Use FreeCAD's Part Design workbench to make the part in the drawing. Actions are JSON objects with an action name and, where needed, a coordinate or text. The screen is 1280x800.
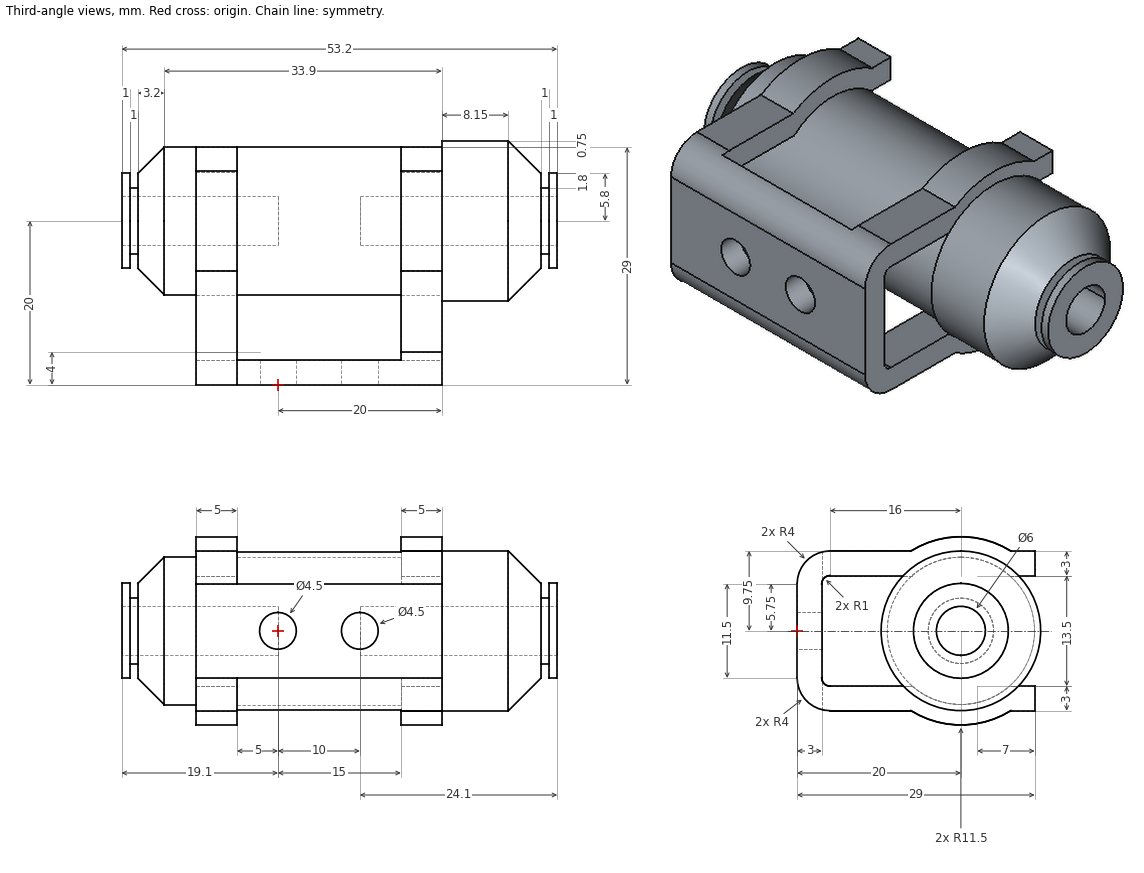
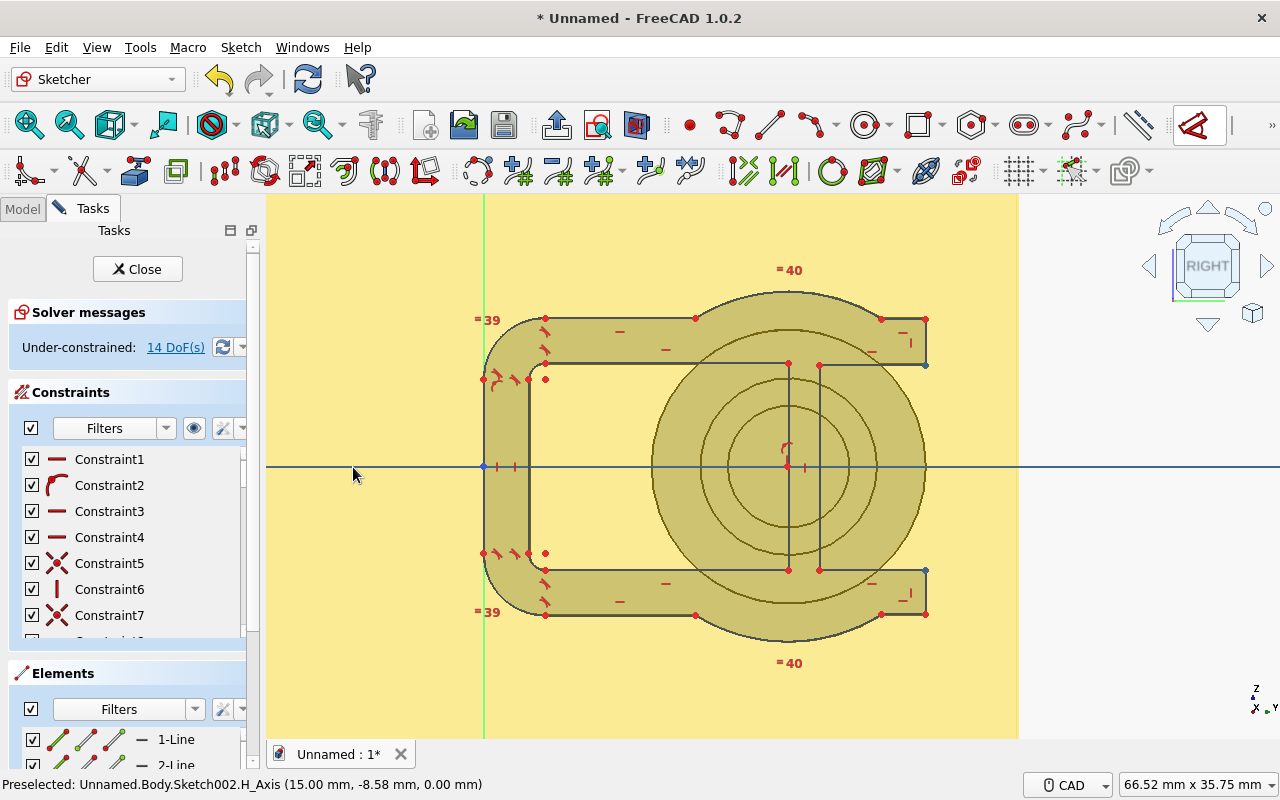
{"action": "key", "text": "s"}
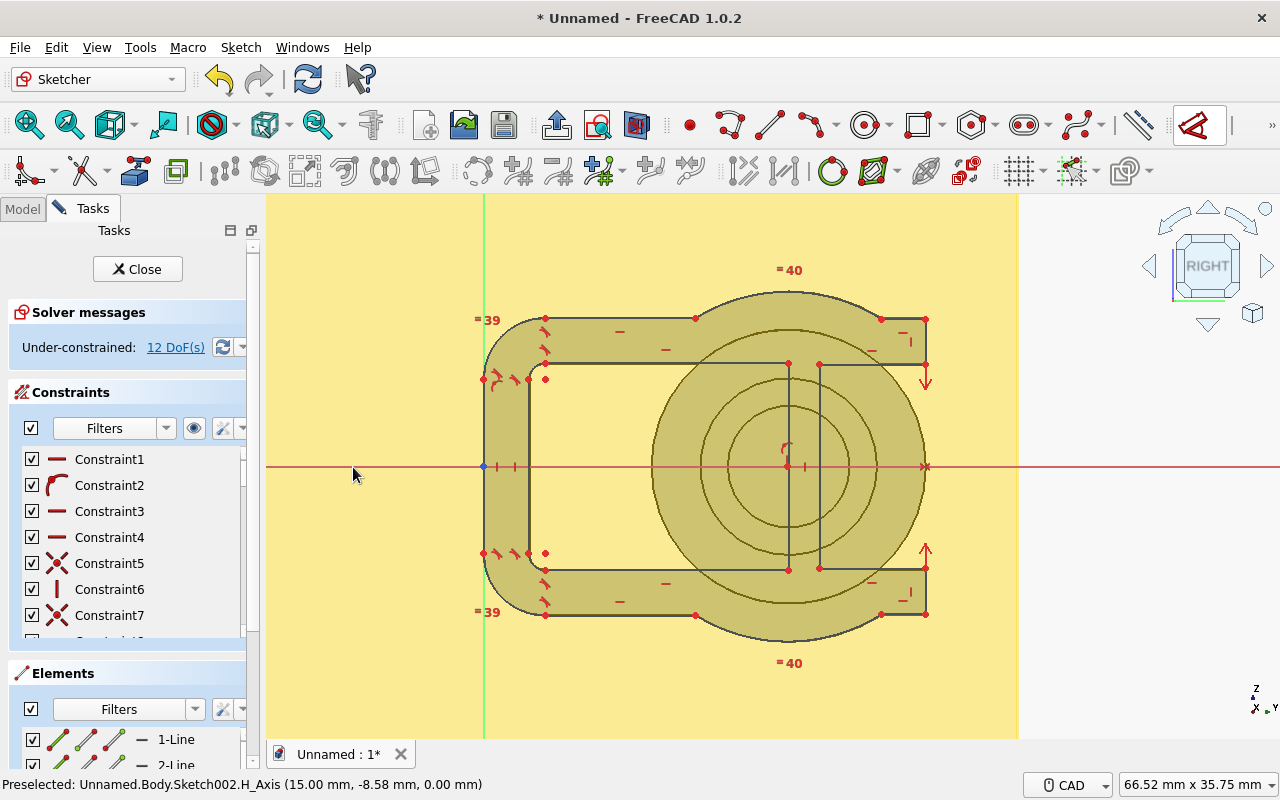
{"action": "left_click", "coordinate": [517, 325]}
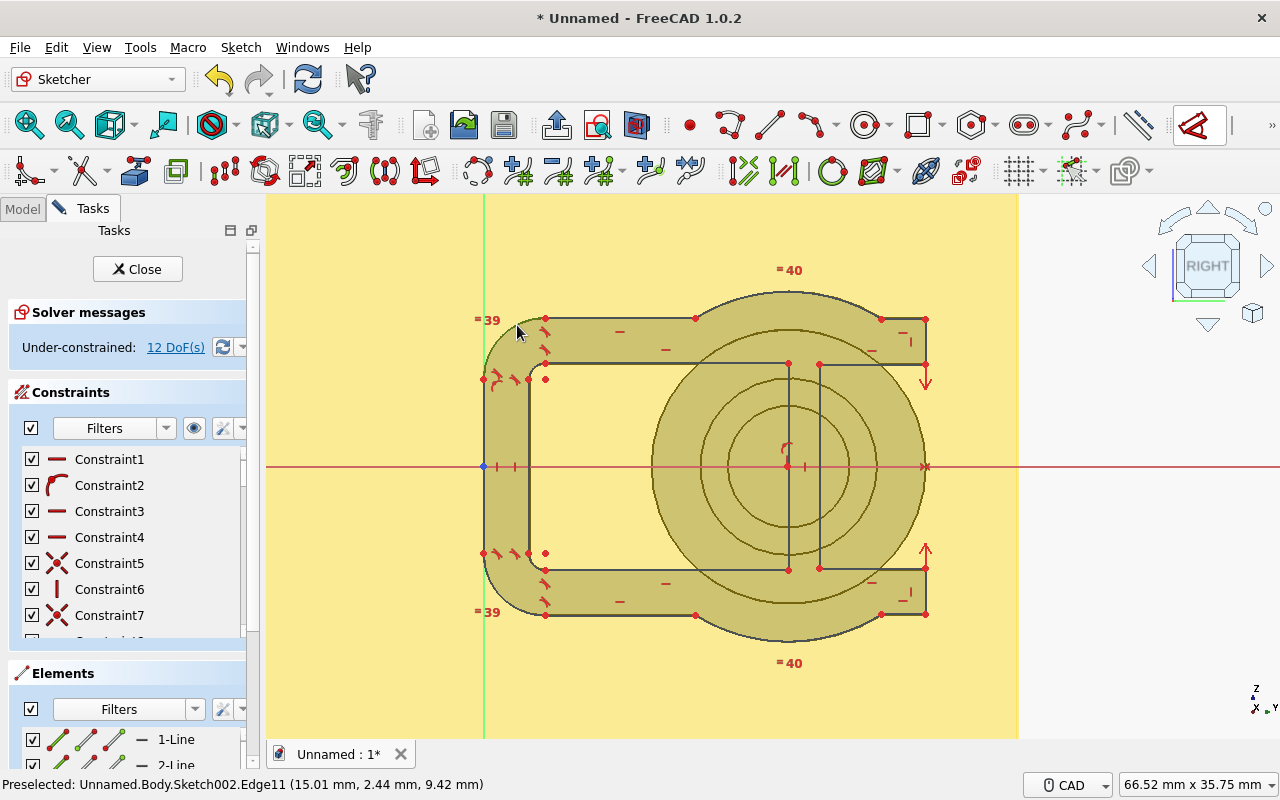
{"action": "left_click", "coordinate": [1220, 126]}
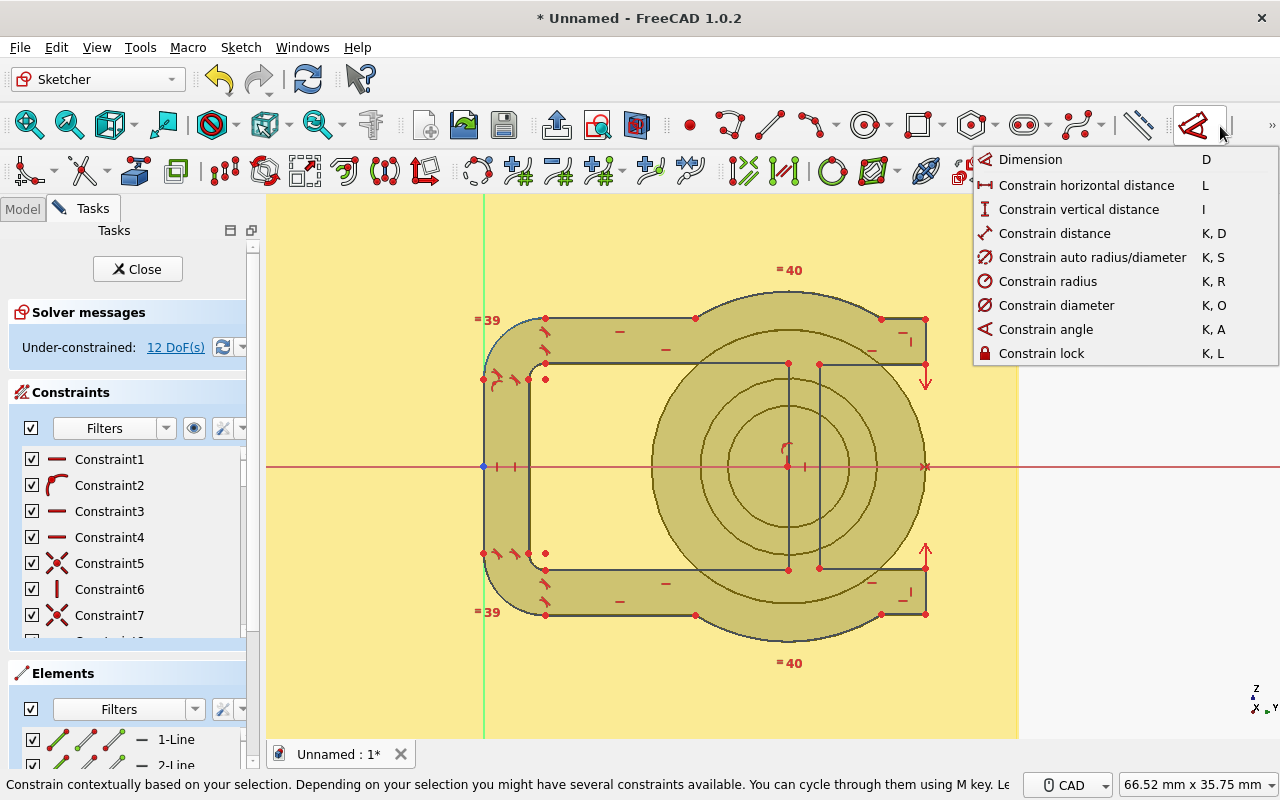
{"action": "left_click", "coordinate": [1126, 281]}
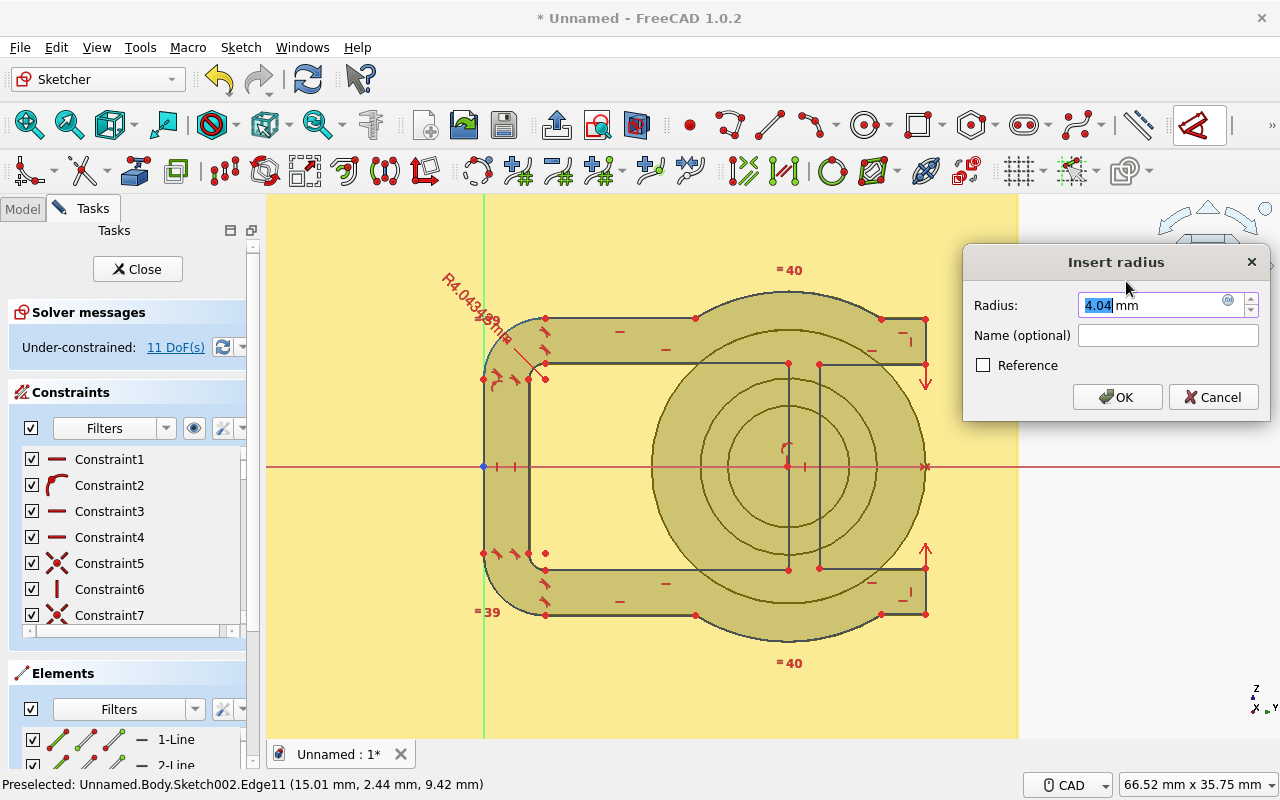
{"action": "type", "text": "4"}
{"action": "key", "text": "Return"}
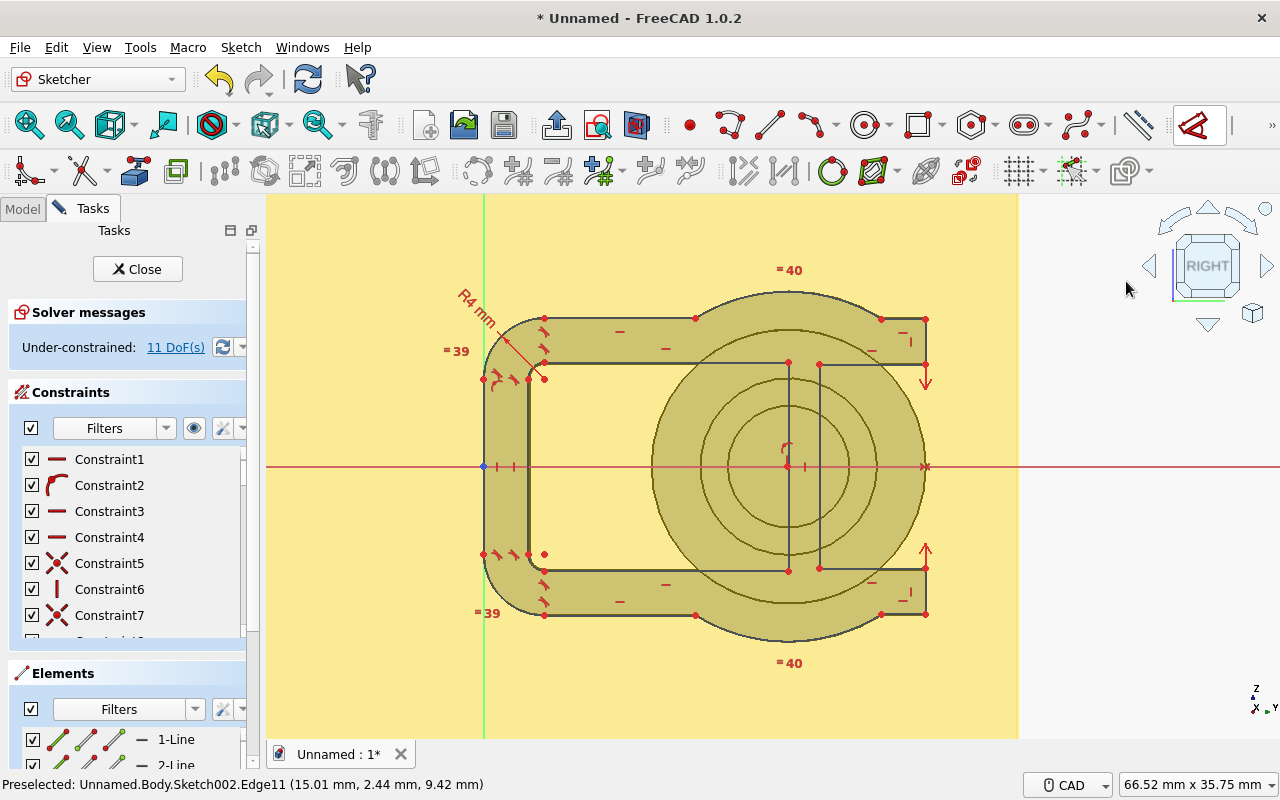
{"action": "left_click", "coordinate": [750, 637]}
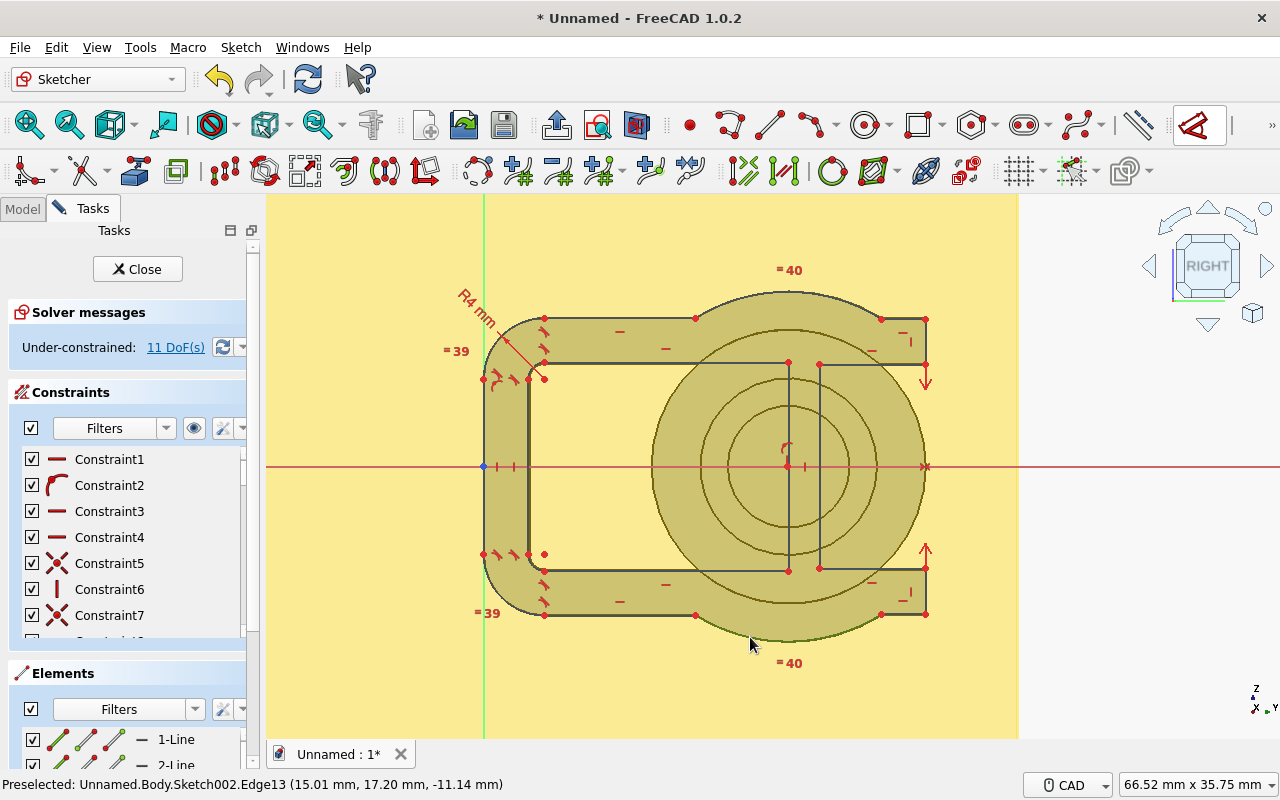
{"action": "key", "text": "k r"}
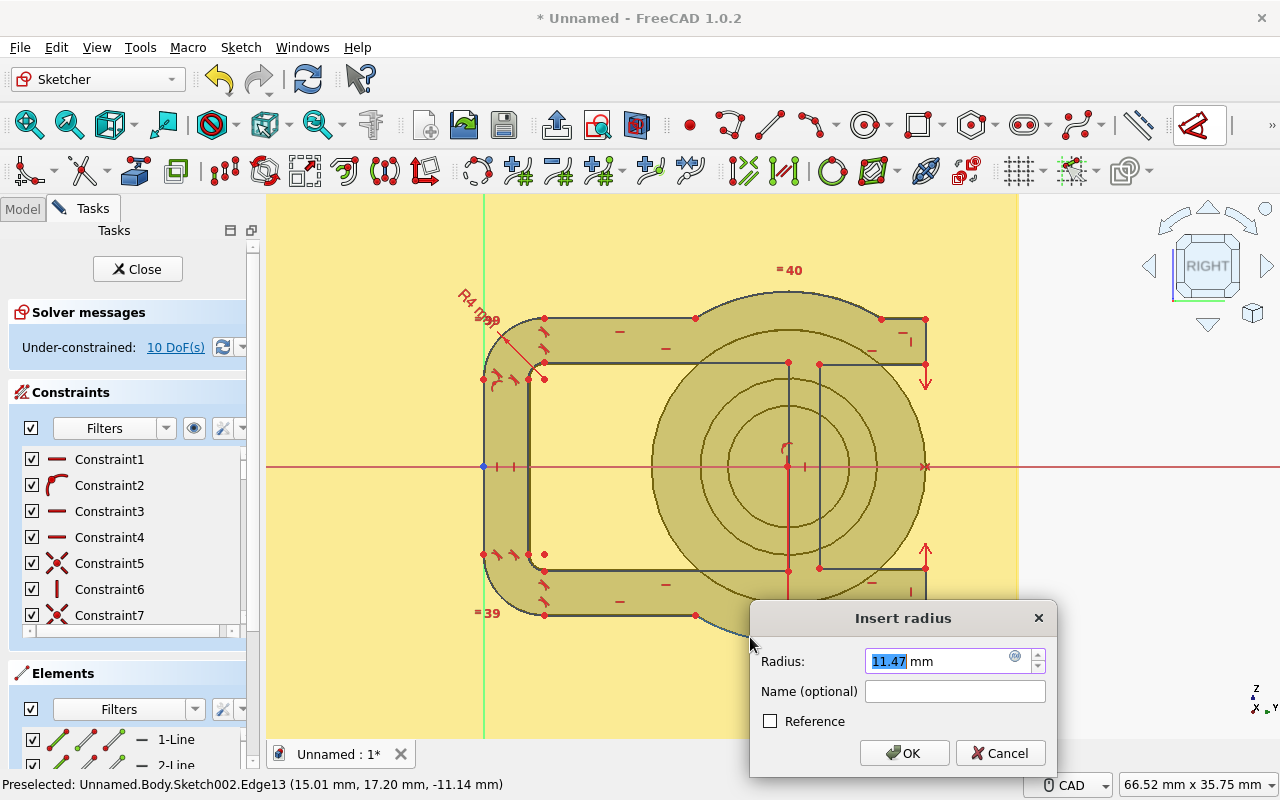
{"action": "type", "text": "11.5"}
{"action": "key", "text": "Return"}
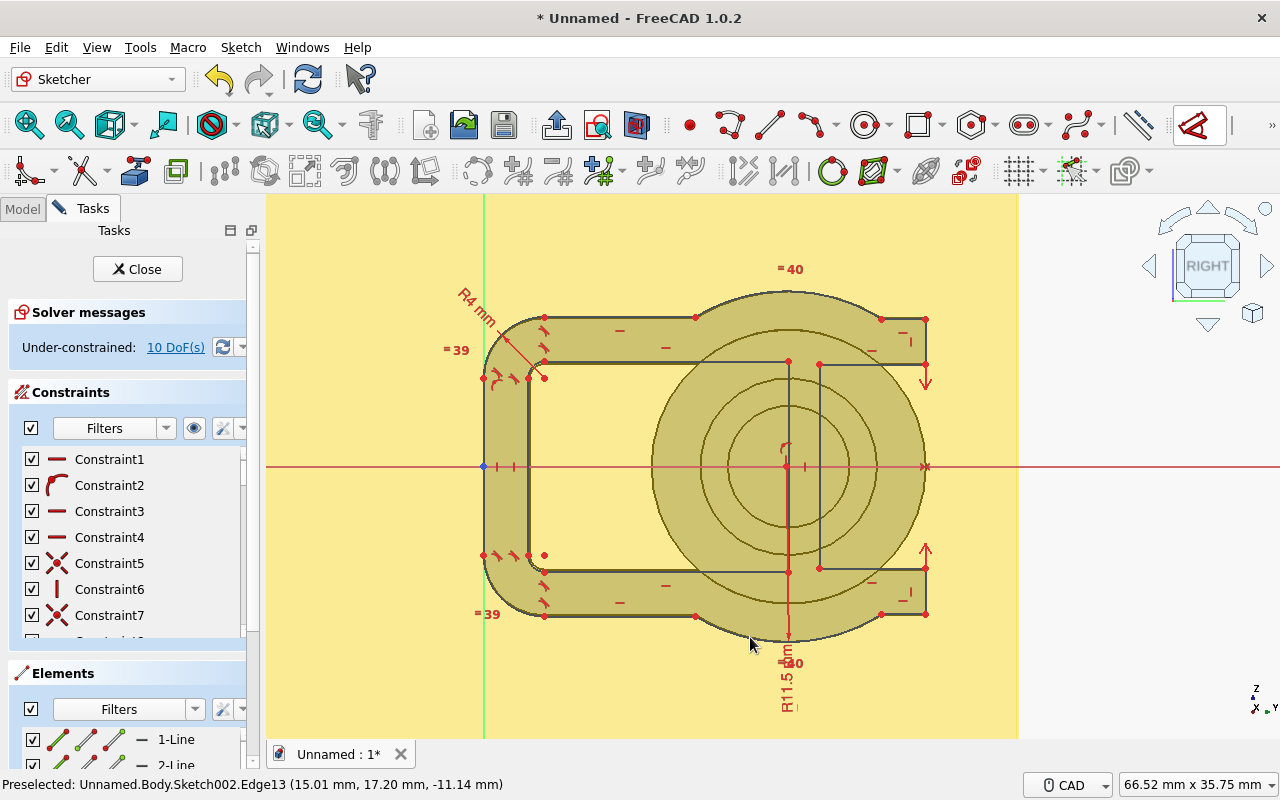
{"action": "scroll", "coordinate": [533, 366], "scroll_direction": "up", "scroll_amount": 5}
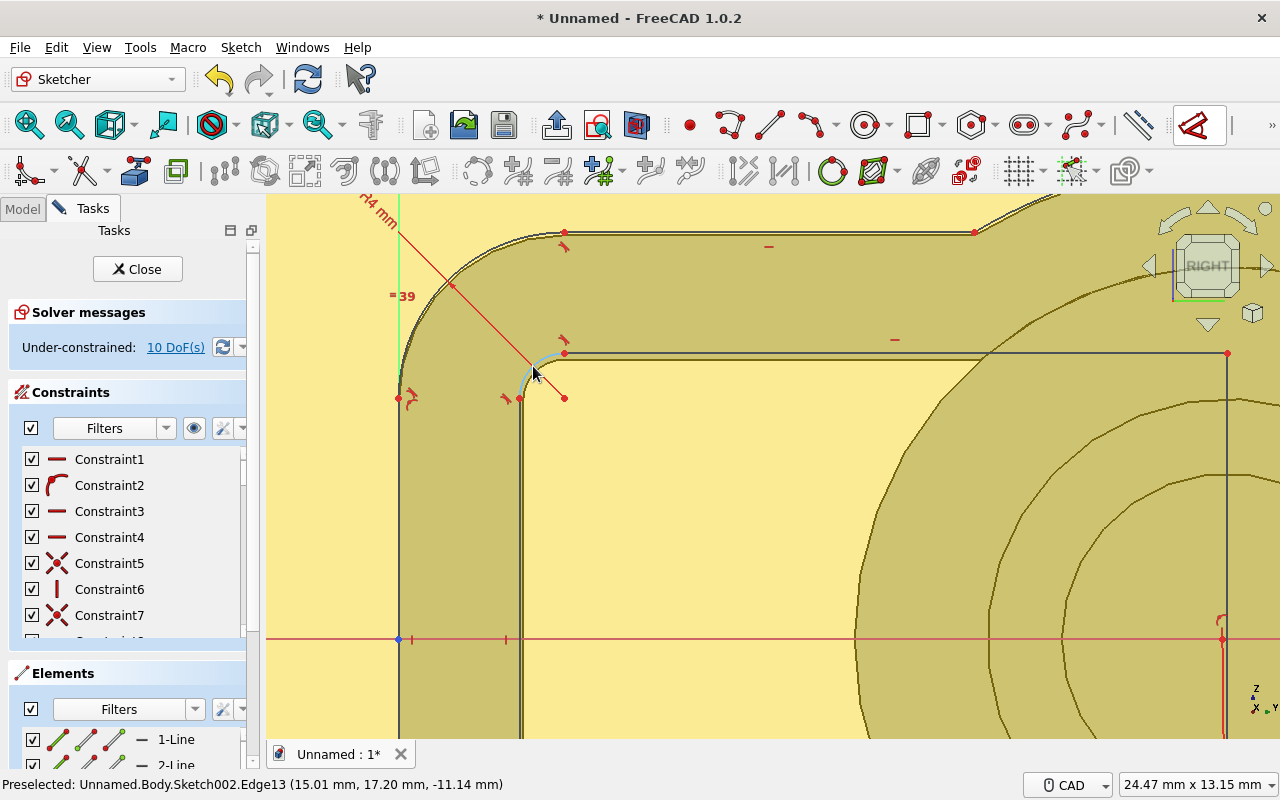
{"action": "left_click", "coordinate": [533, 367]}